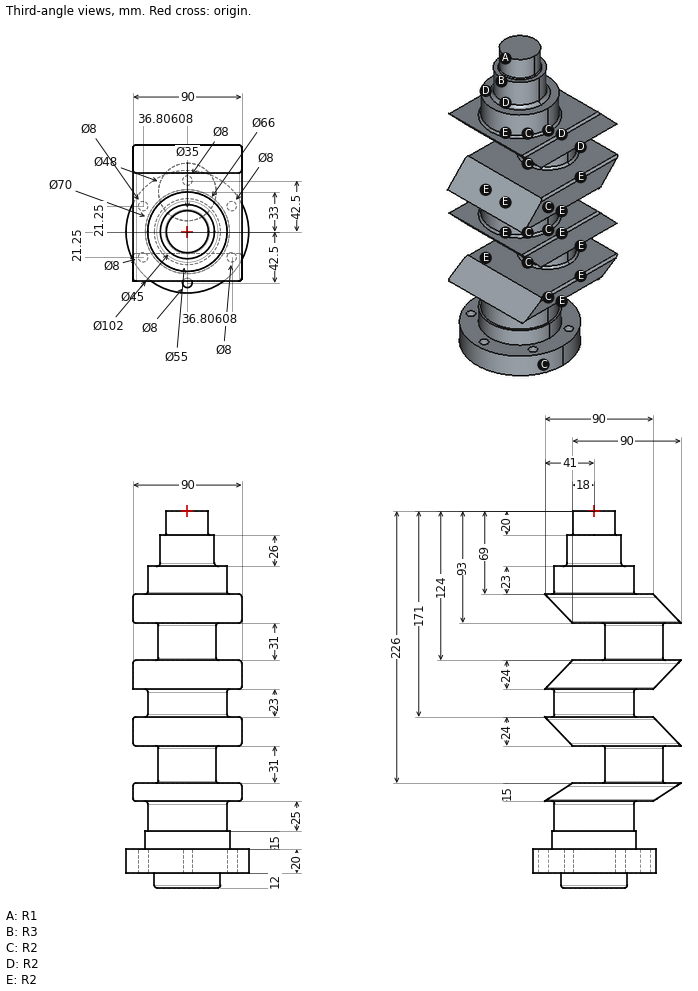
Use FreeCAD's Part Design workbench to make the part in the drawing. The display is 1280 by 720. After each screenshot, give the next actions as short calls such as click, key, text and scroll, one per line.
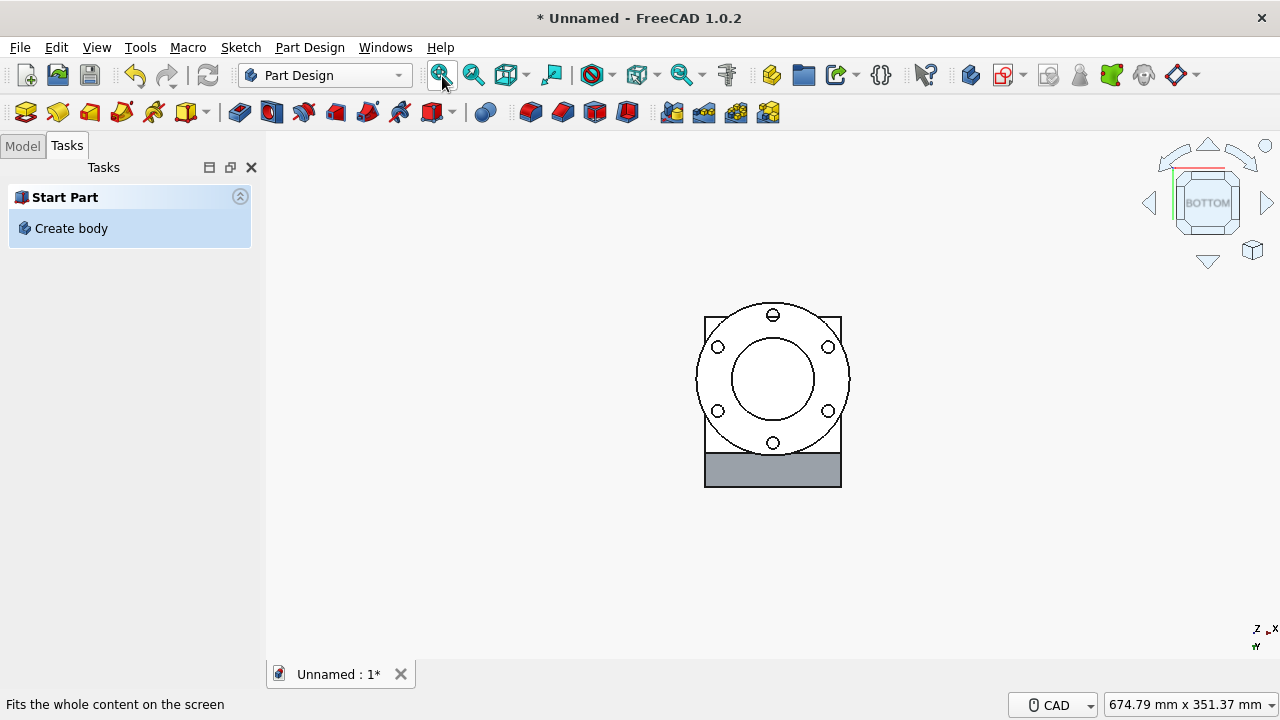
click(442, 76)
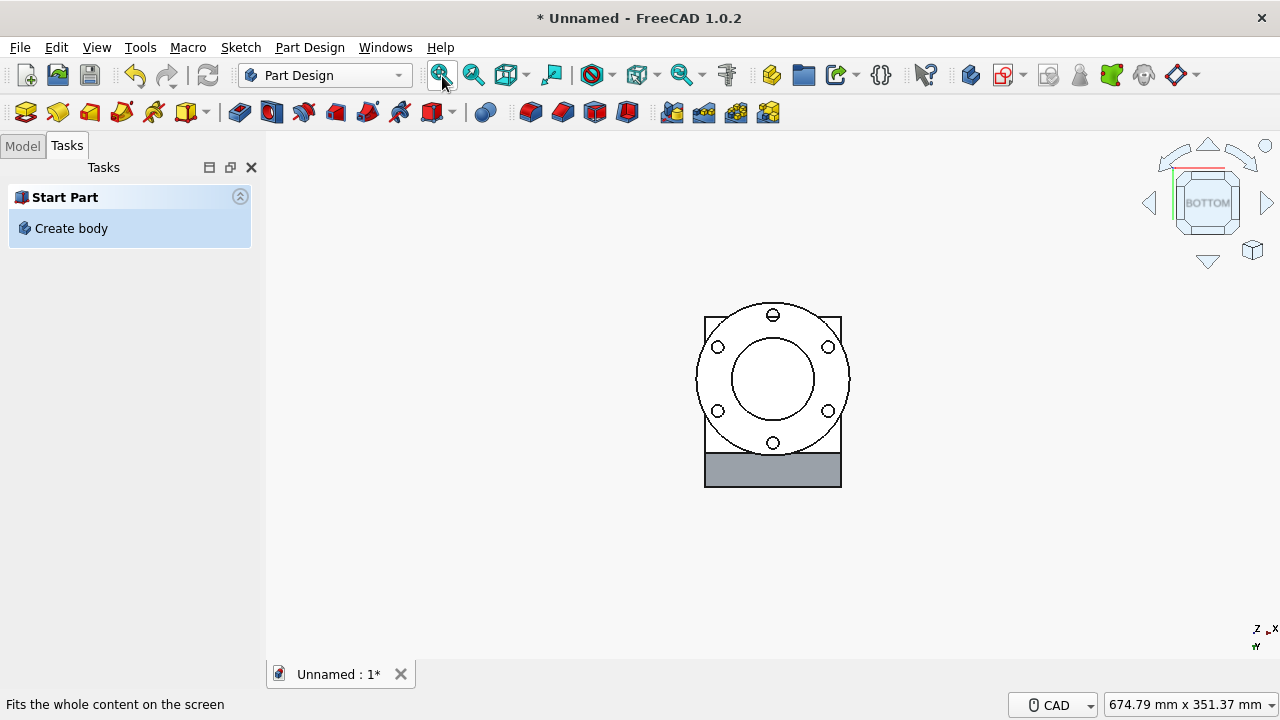
key(4)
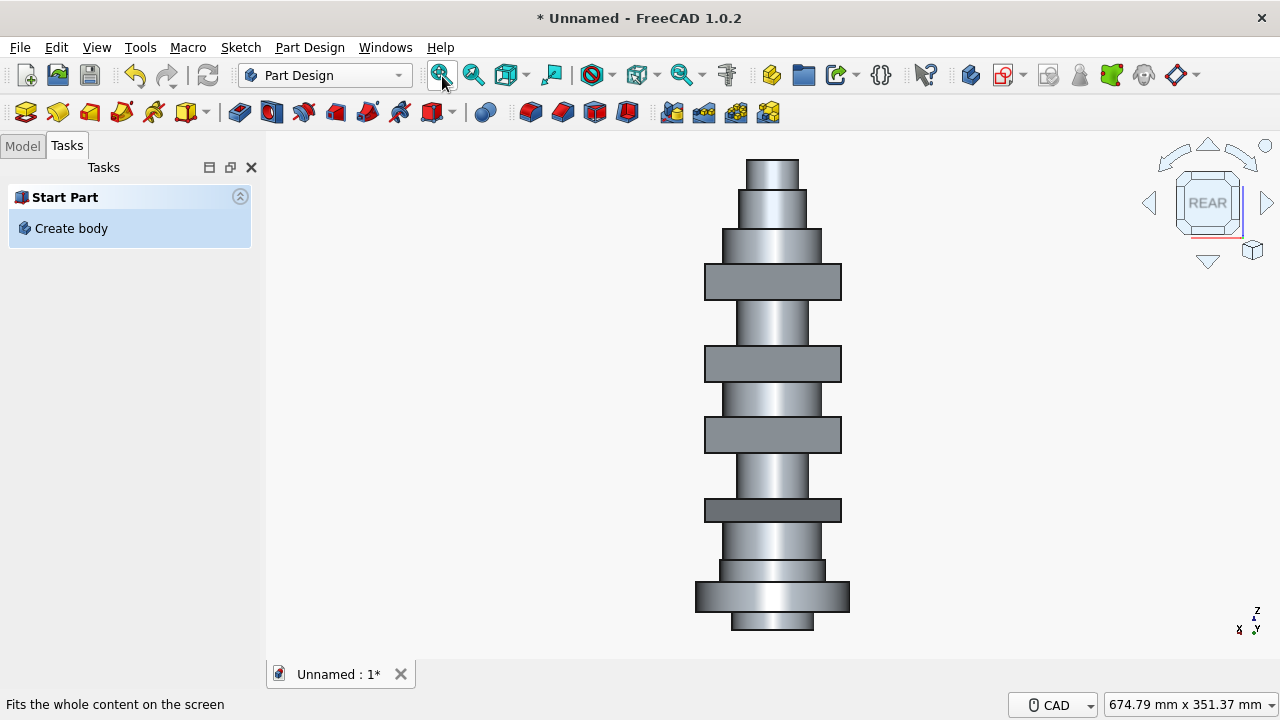
key(6)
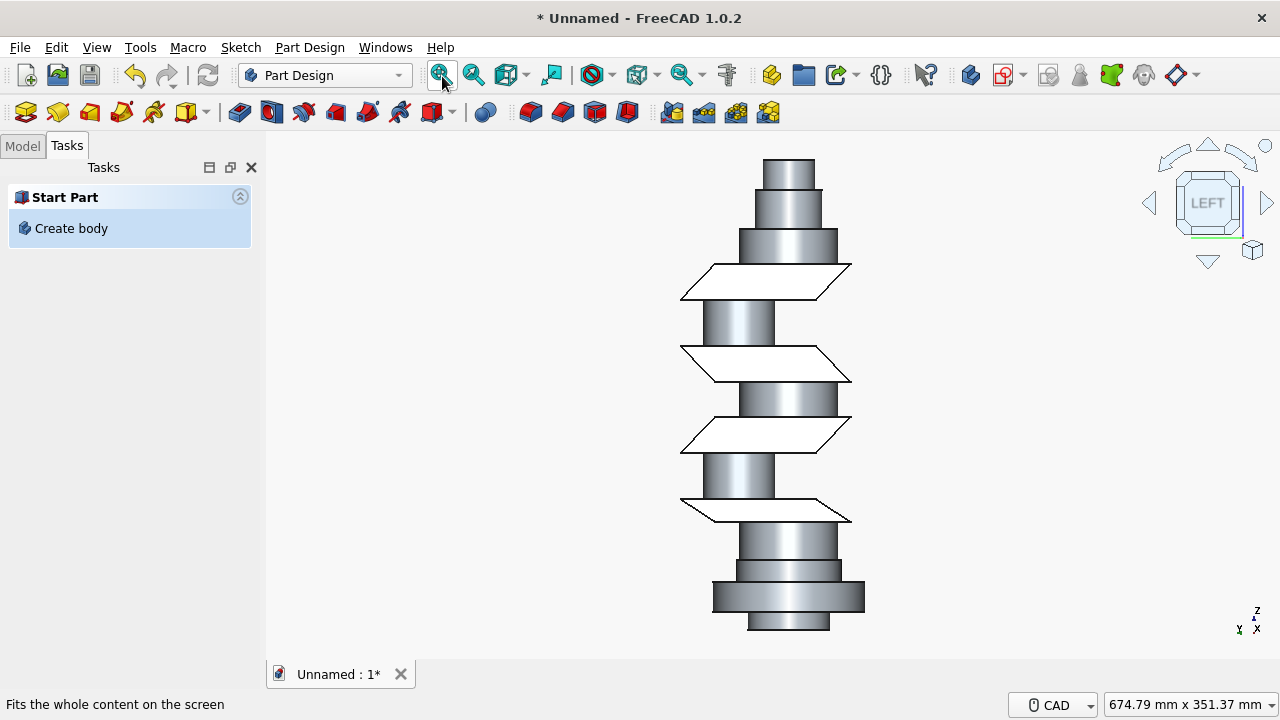
key(v)
key(3)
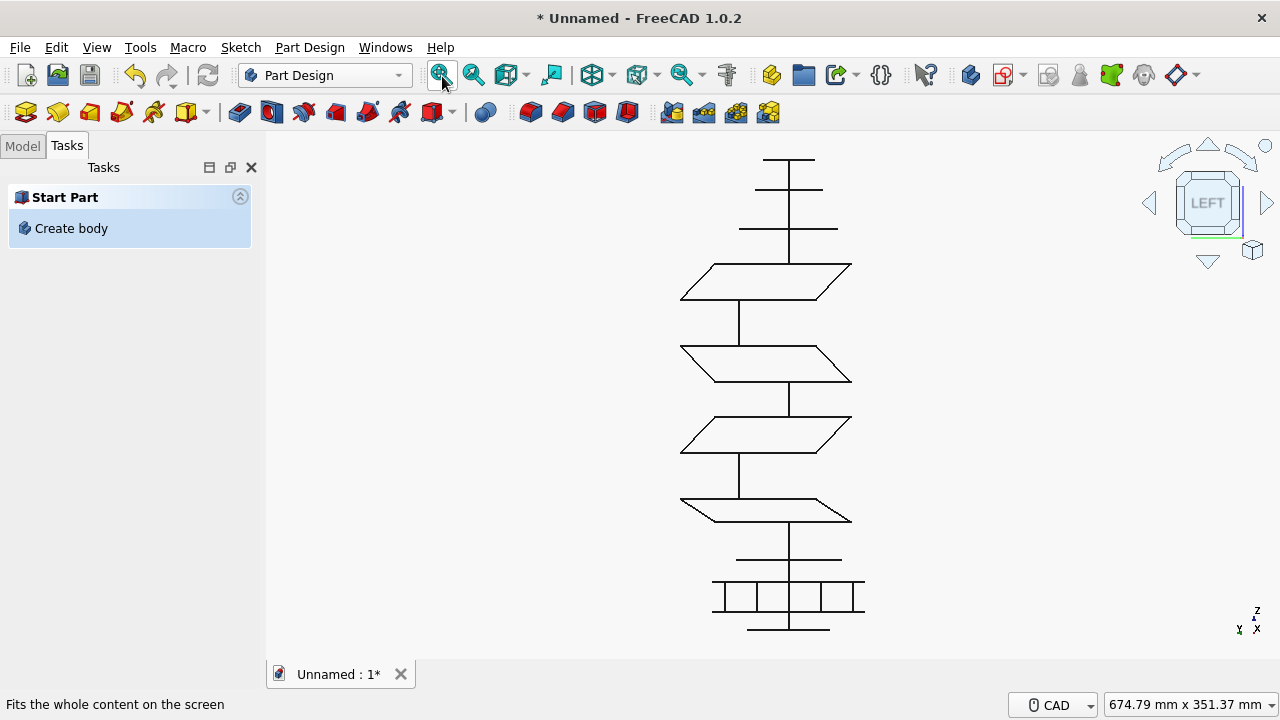
key(0)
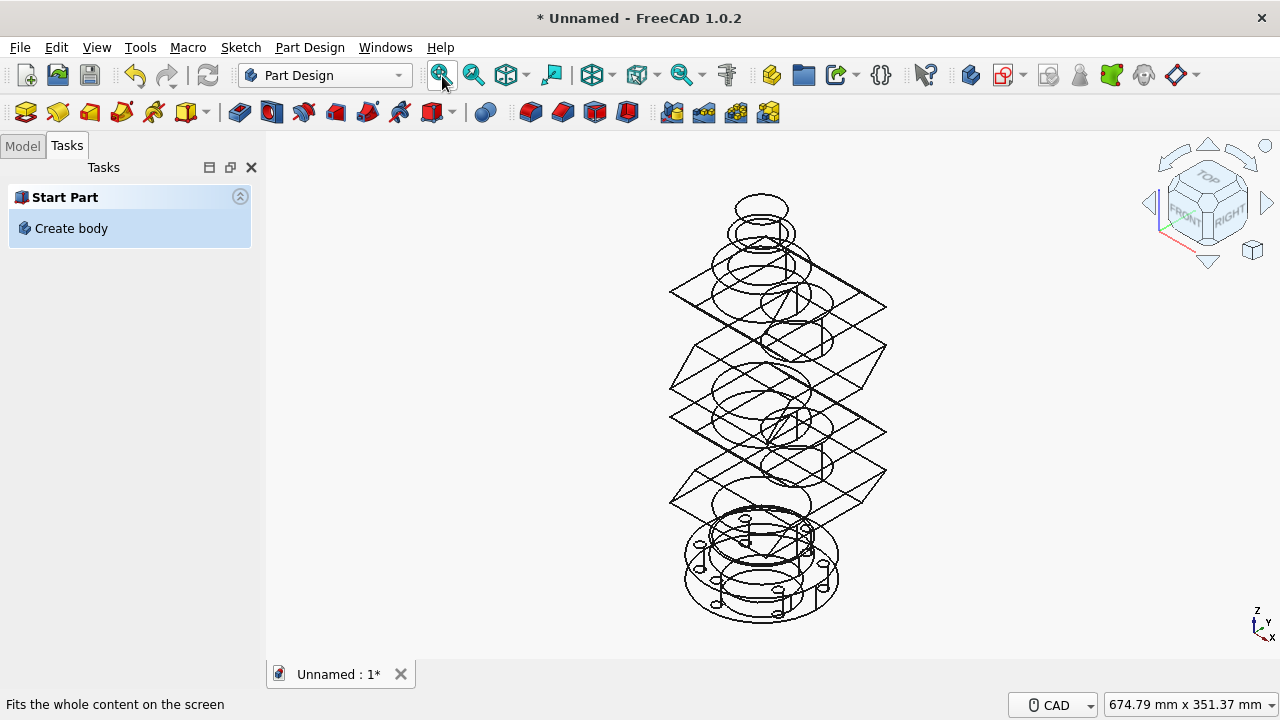
click(736, 231)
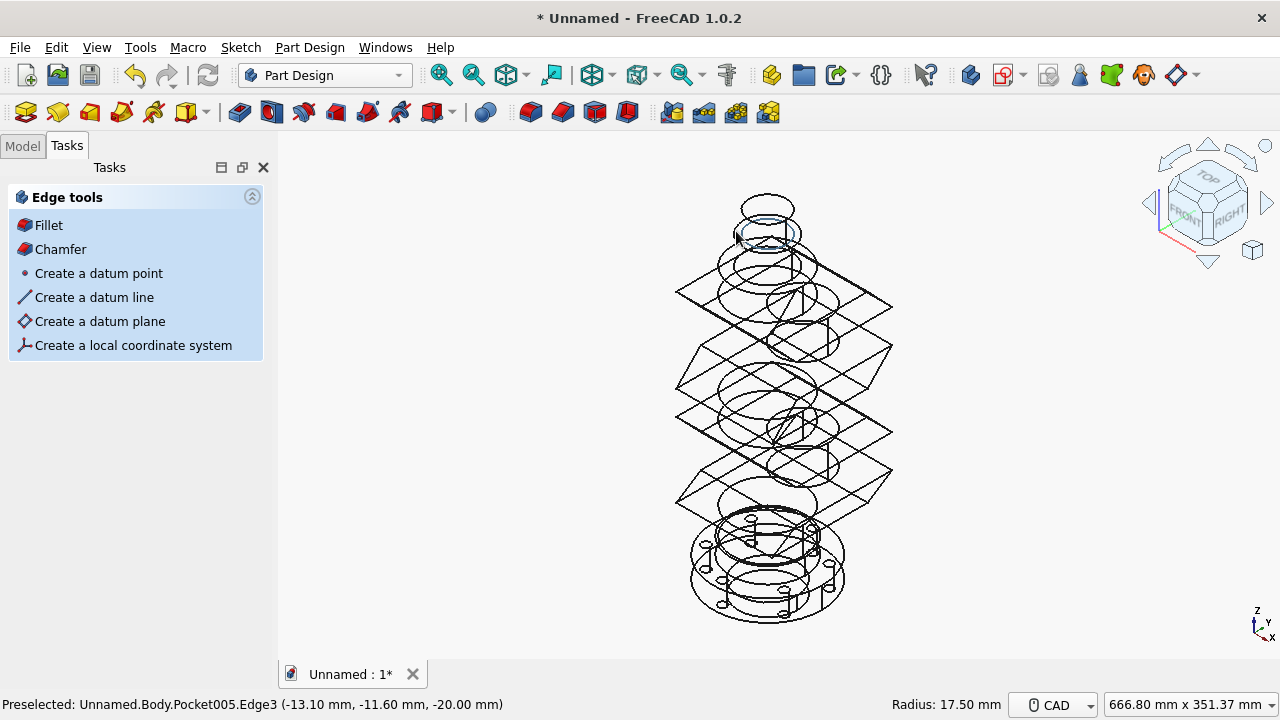
key(v)
key(1)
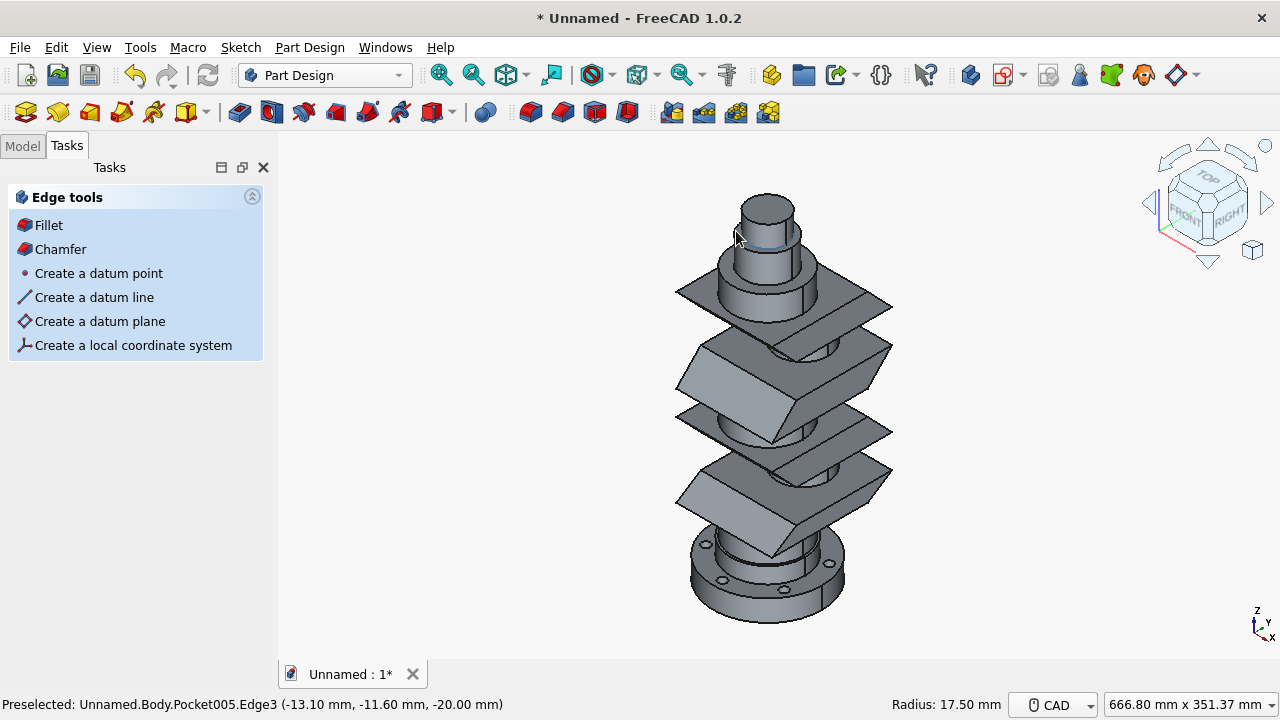
click(532, 112)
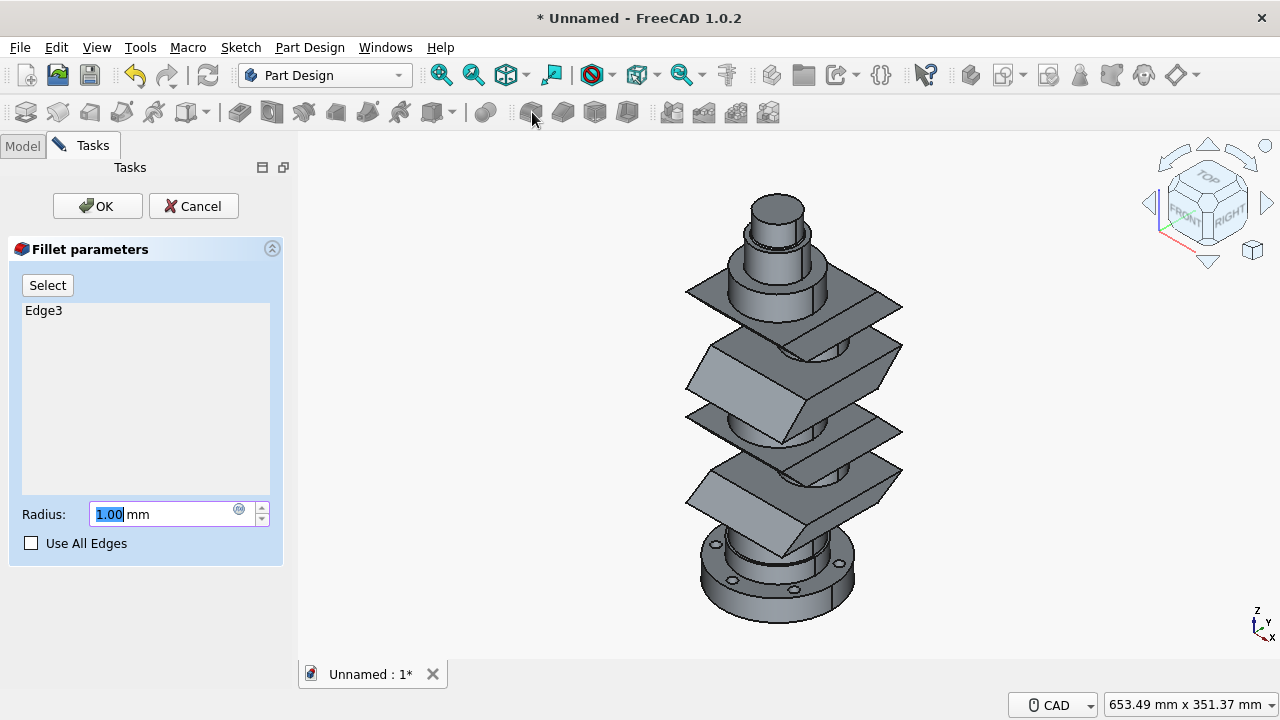
text(1)
key(Tab)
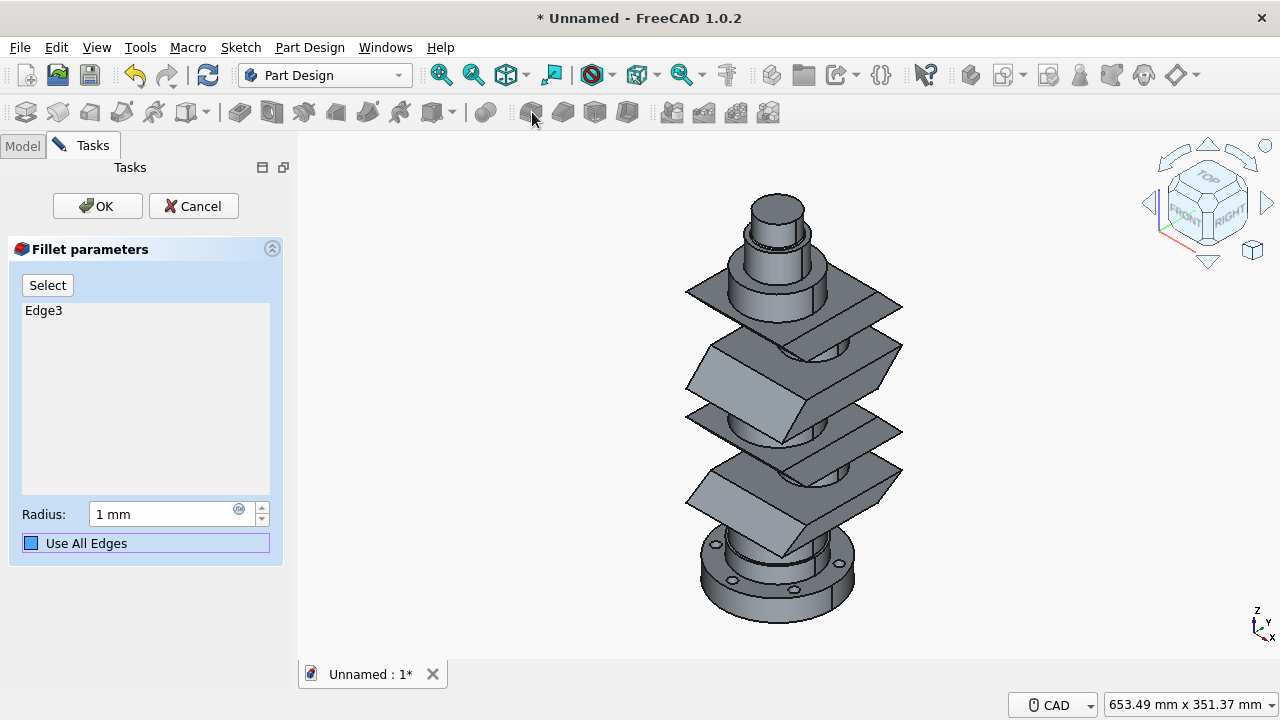
click(98, 206)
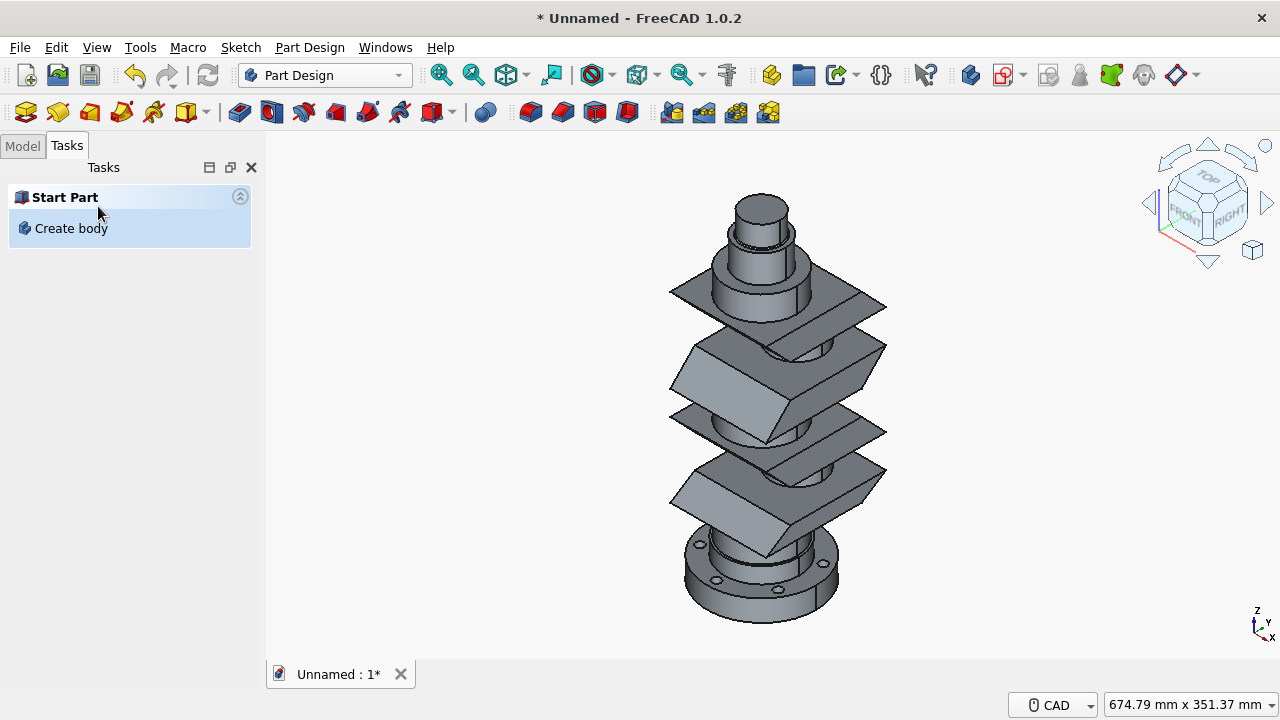
key(2)